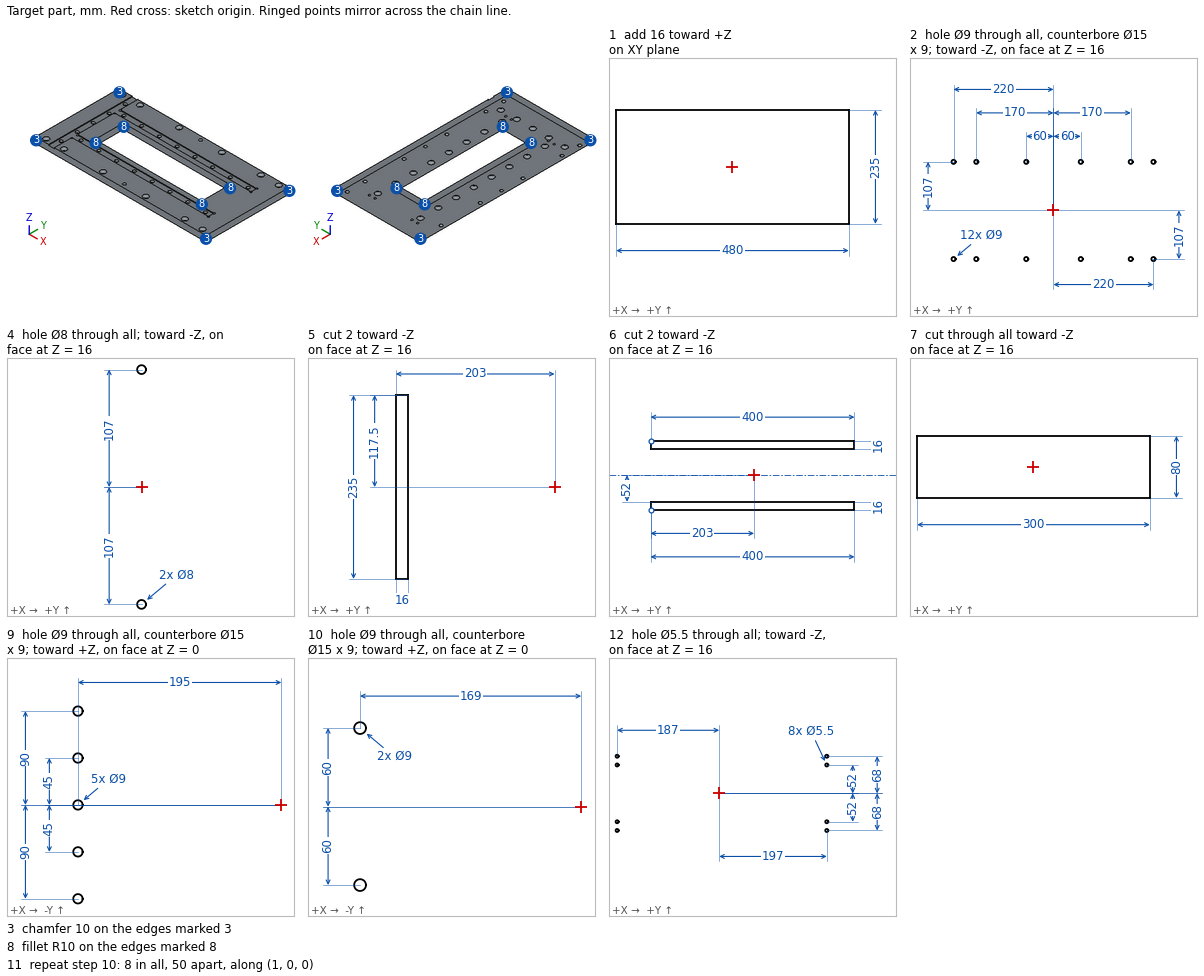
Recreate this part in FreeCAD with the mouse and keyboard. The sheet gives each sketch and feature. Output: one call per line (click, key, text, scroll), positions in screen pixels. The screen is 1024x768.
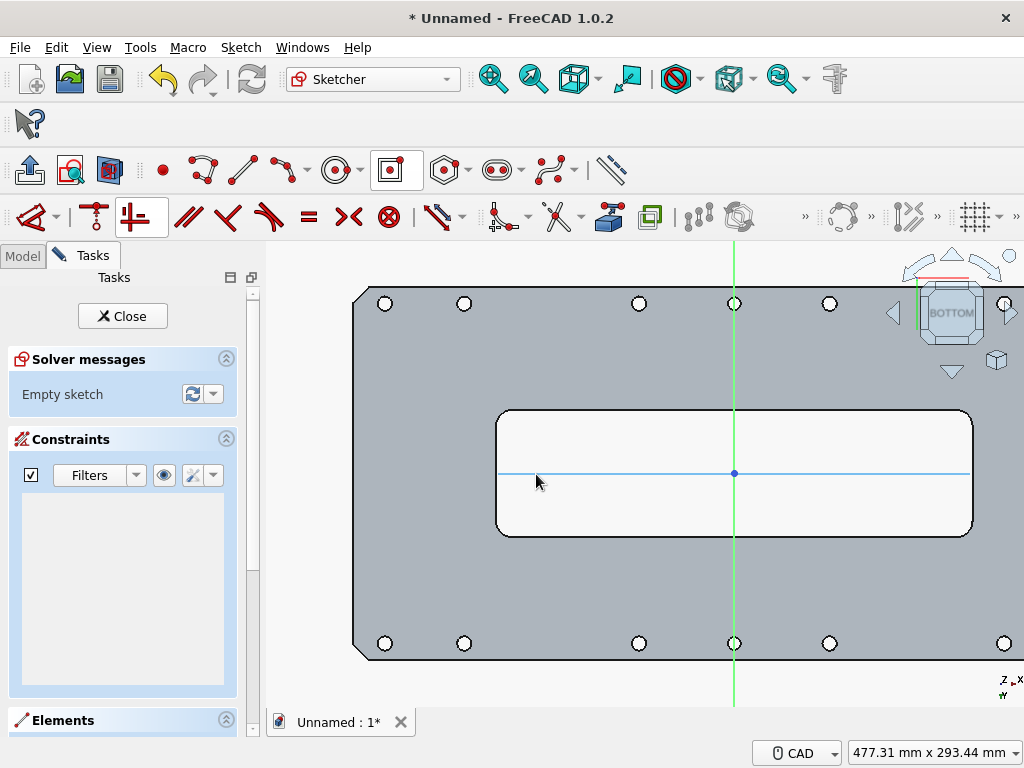
click(336, 170)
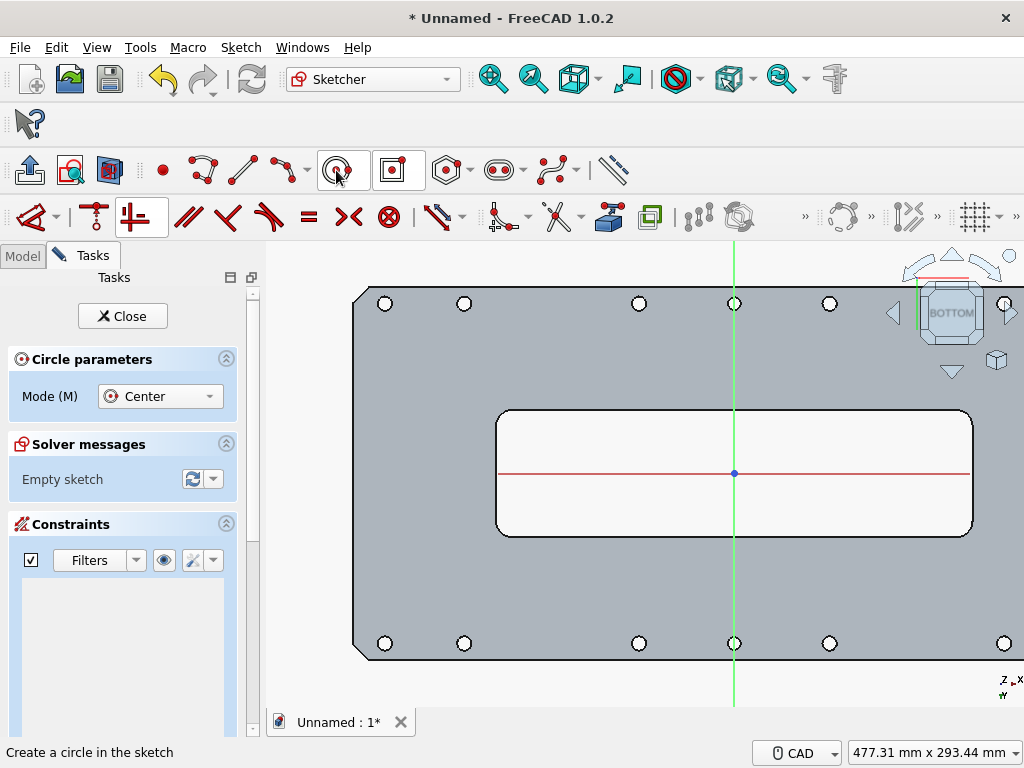
scroll(425, 474, up, 6)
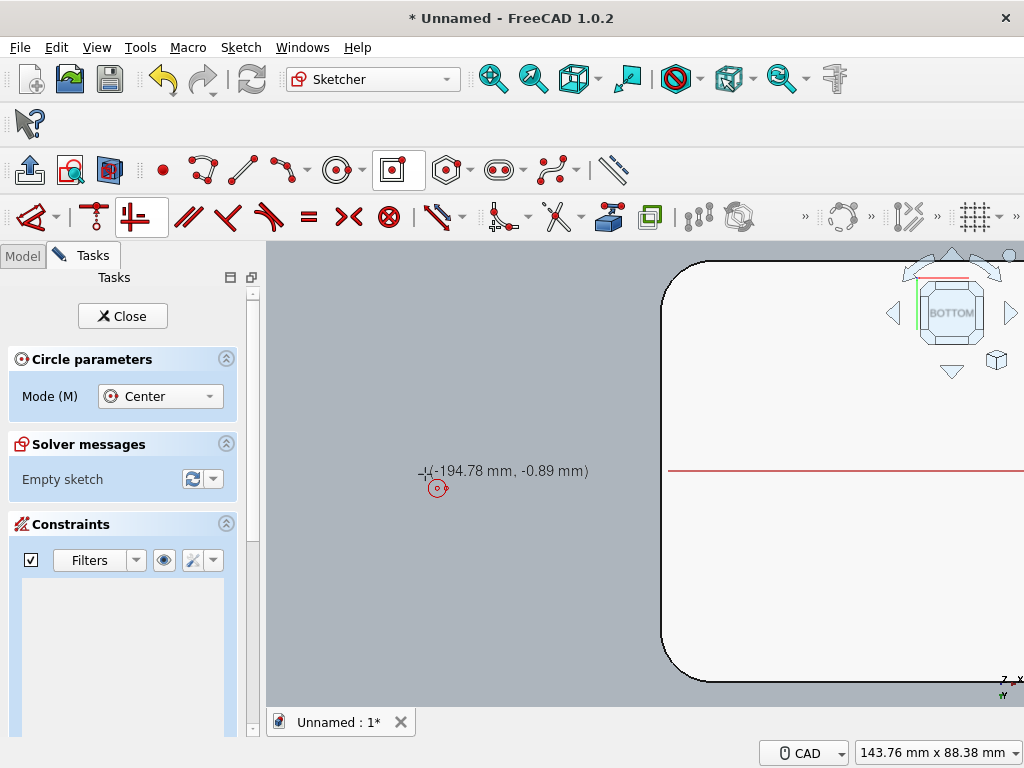
click(423, 471)
move(440, 455)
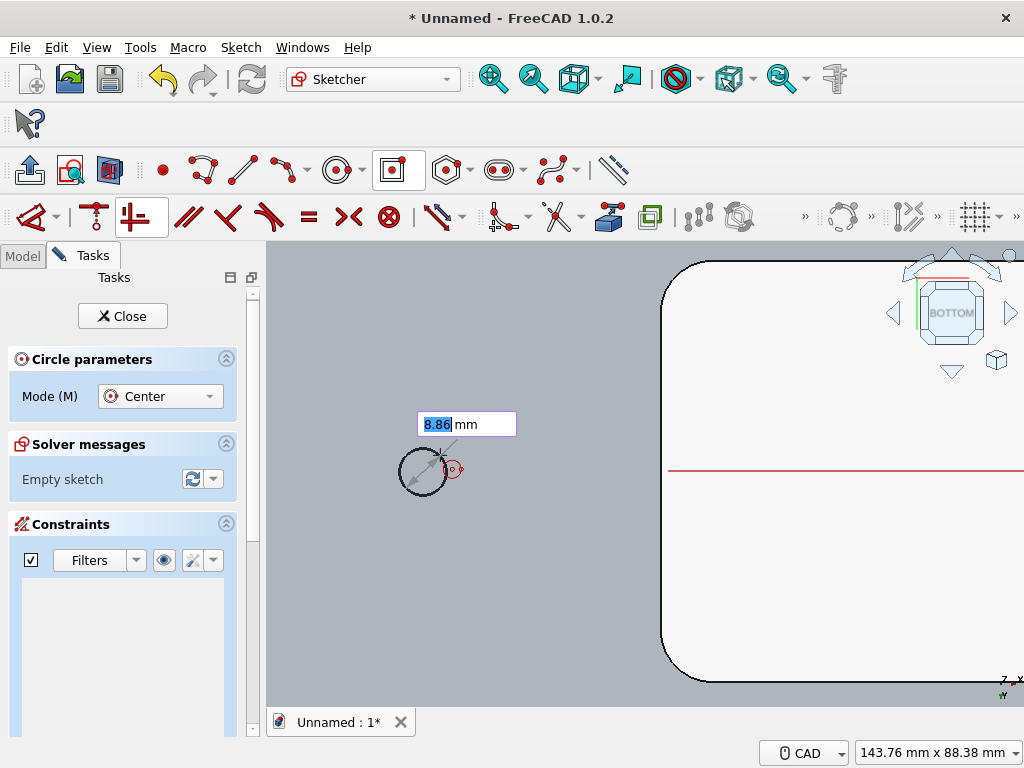
text(9)
key(Return)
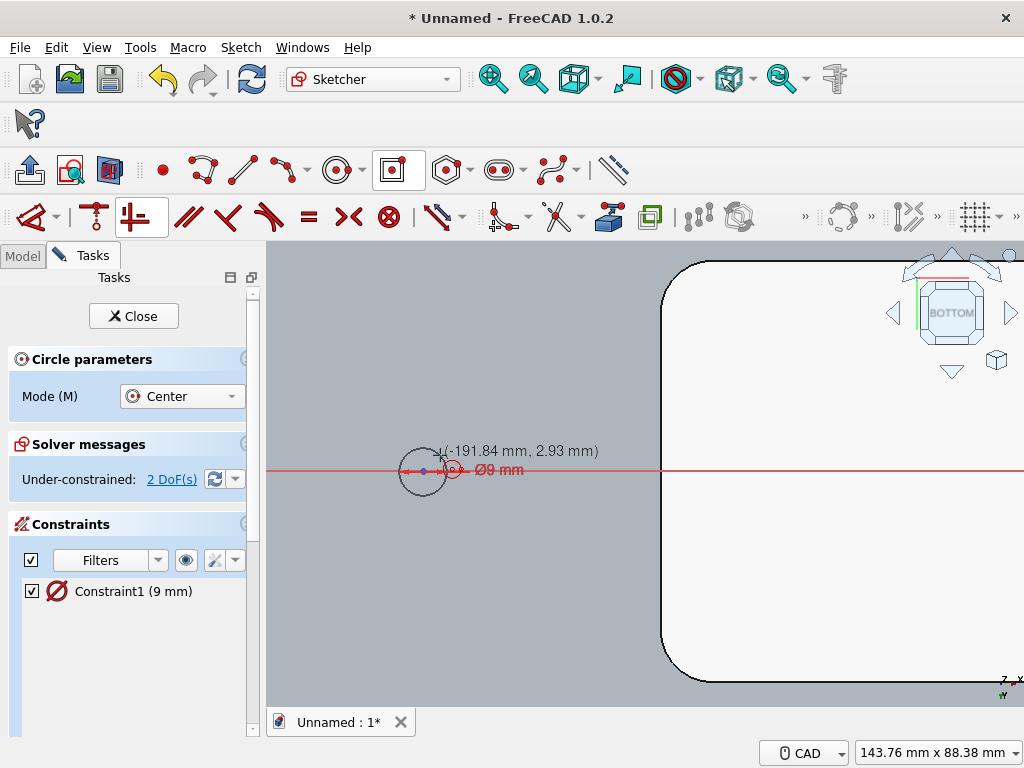
scroll(426, 475, down, 6)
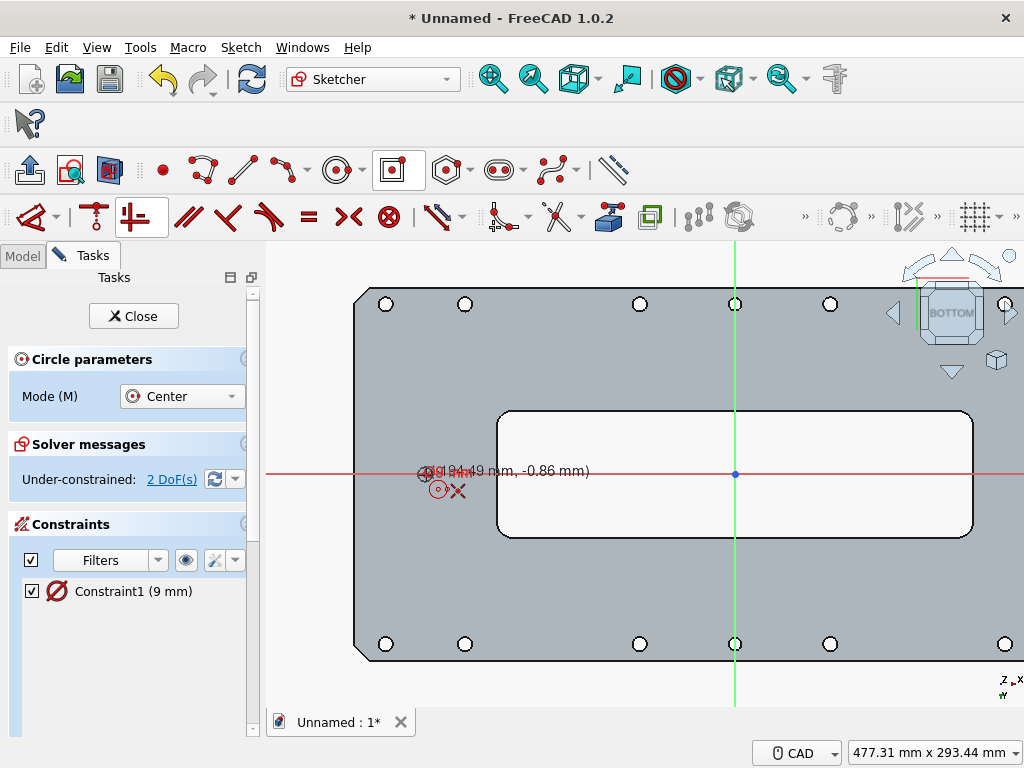
scroll(425, 546, up, 6)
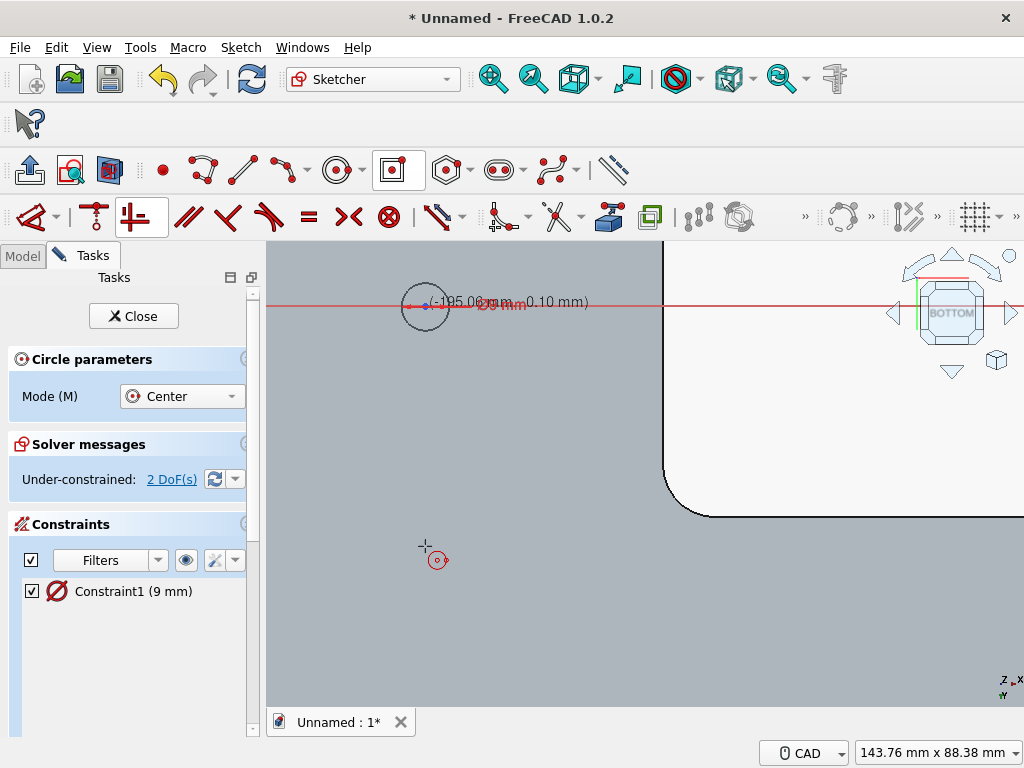
click(426, 544)
move(442, 527)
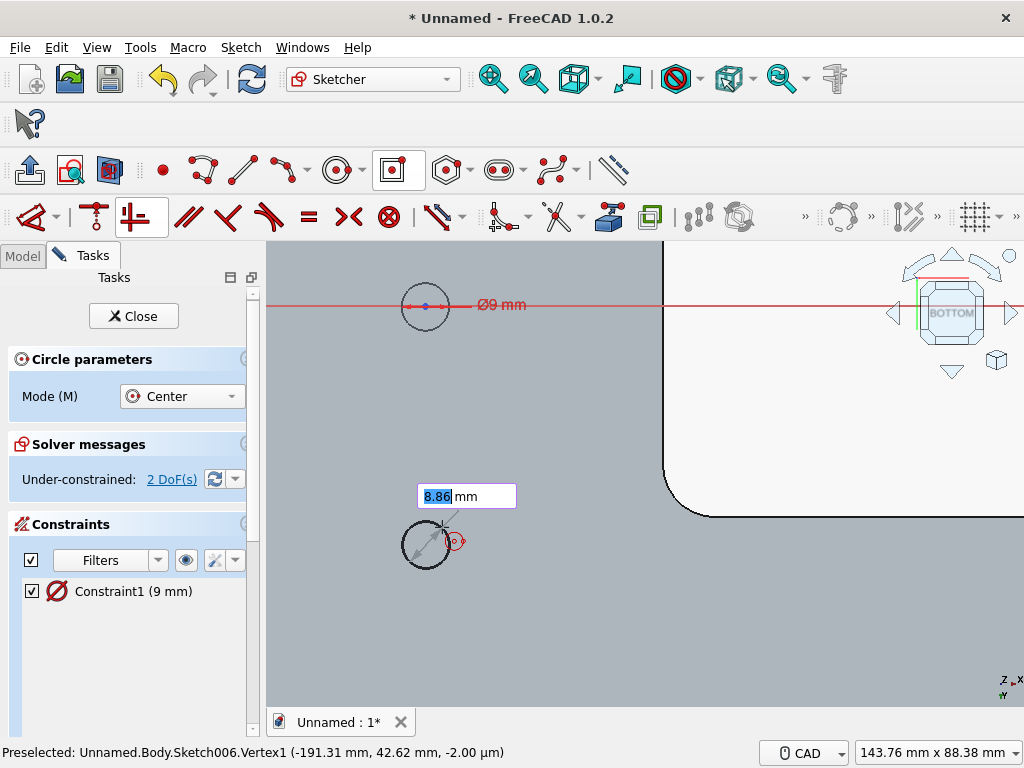
text(9)
key(Return)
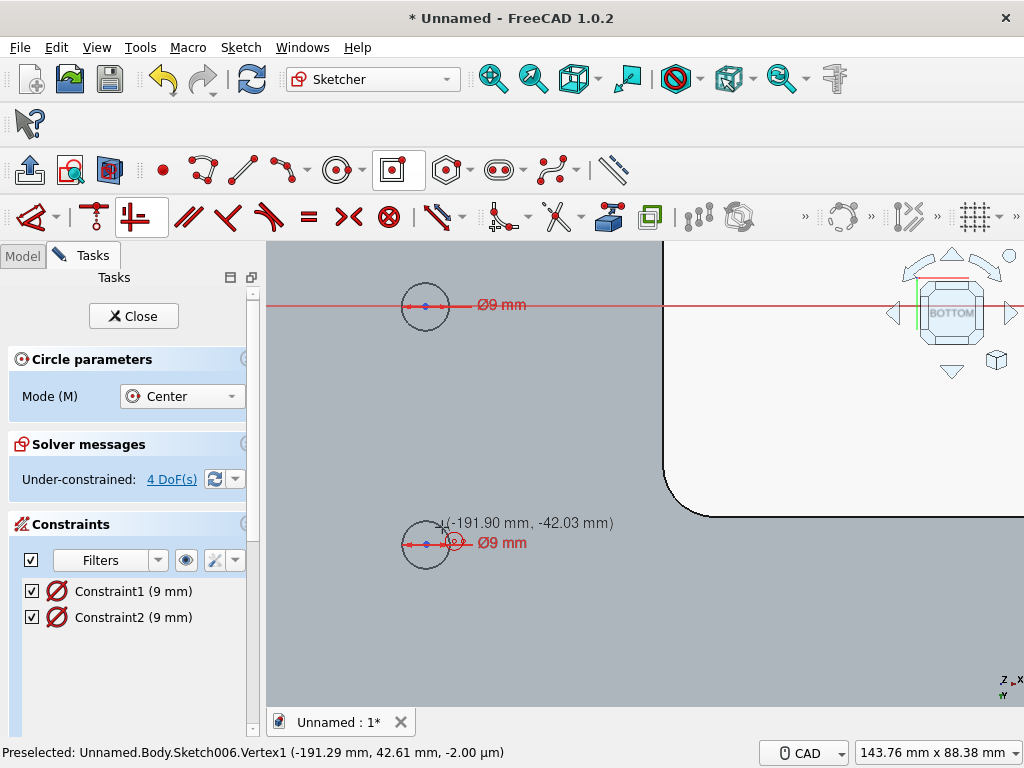
scroll(425, 546, down, 6)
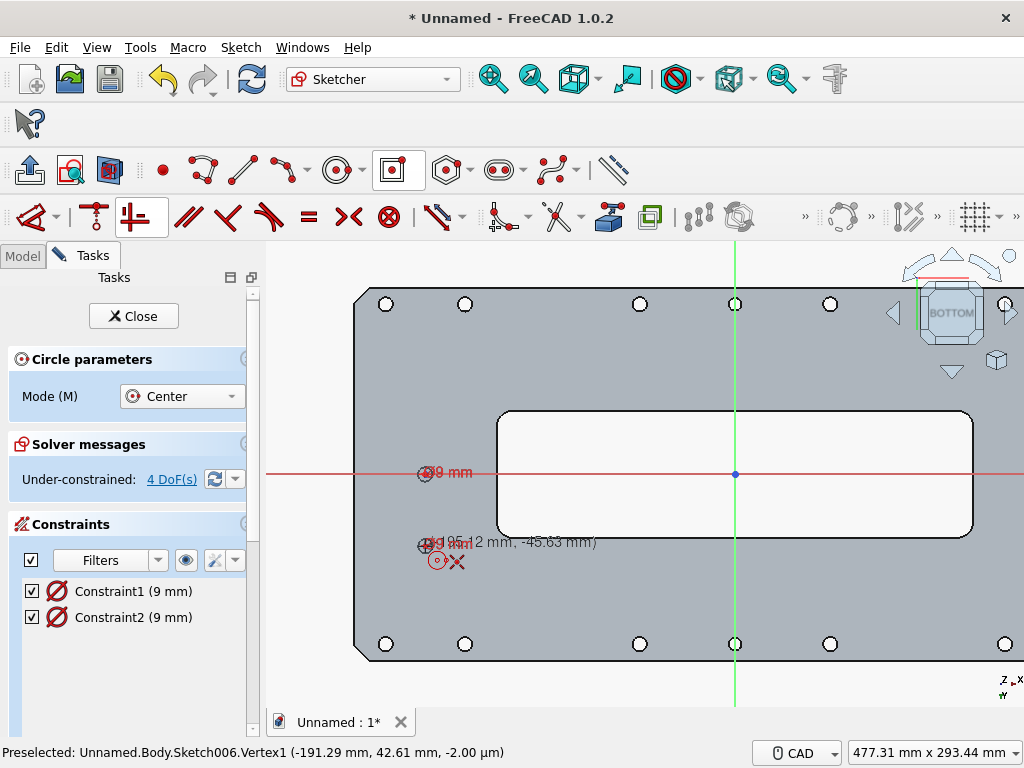
scroll(425, 617, up, 6)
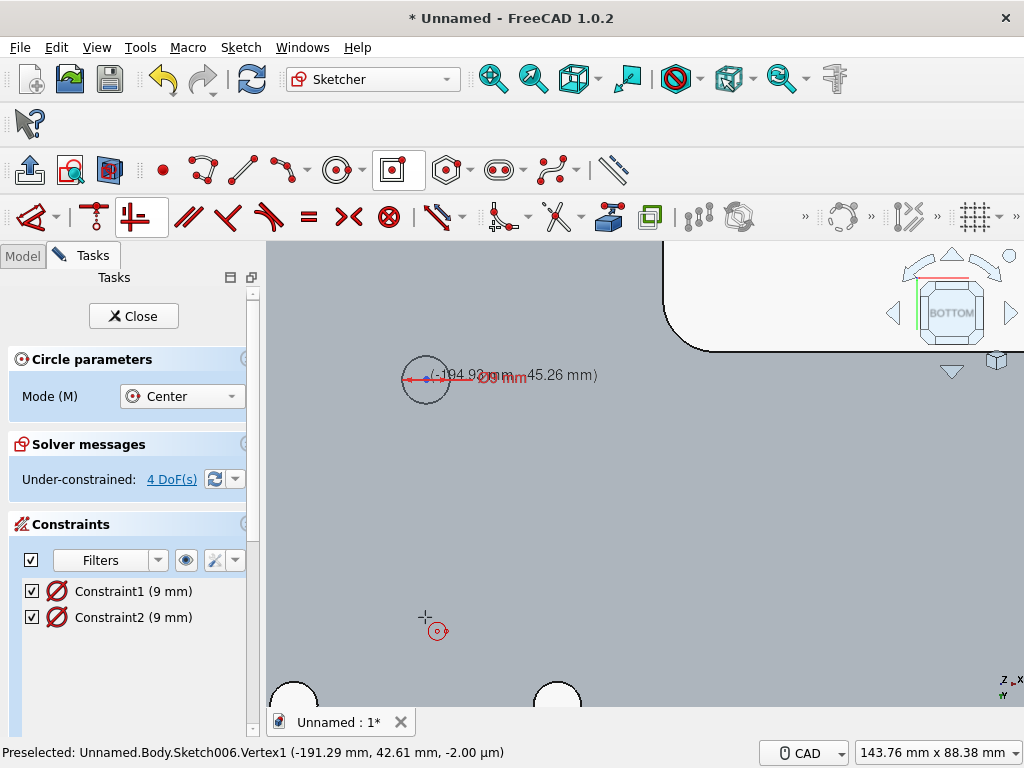
click(426, 616)
move(442, 599)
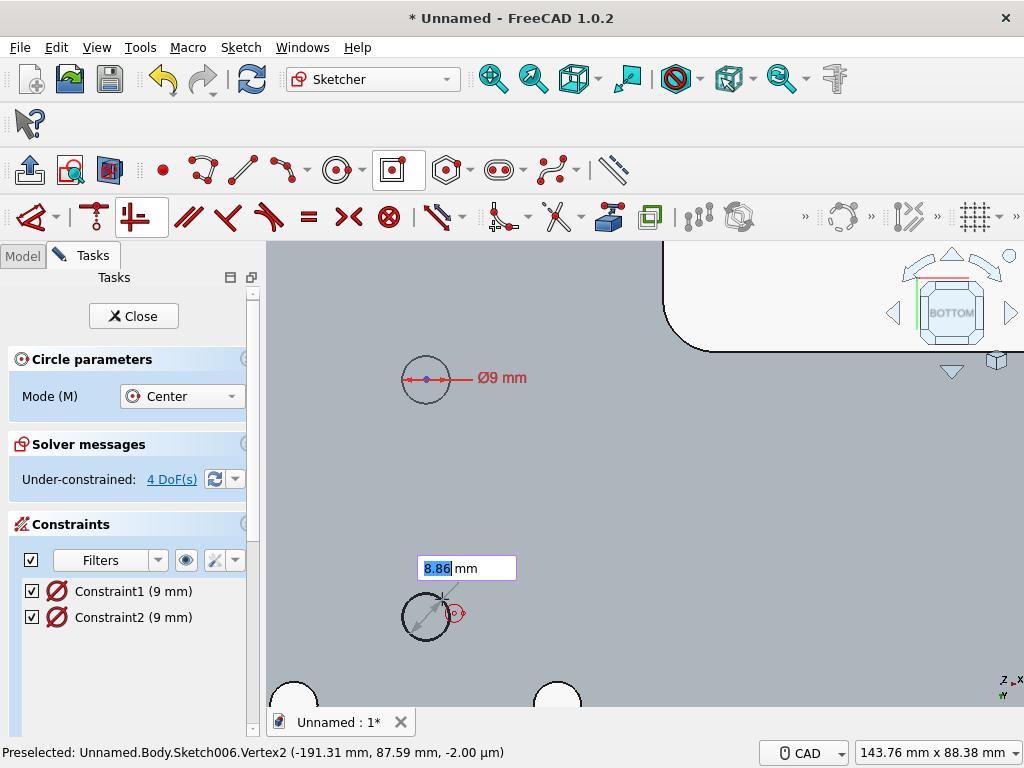
text(9)
key(Return)